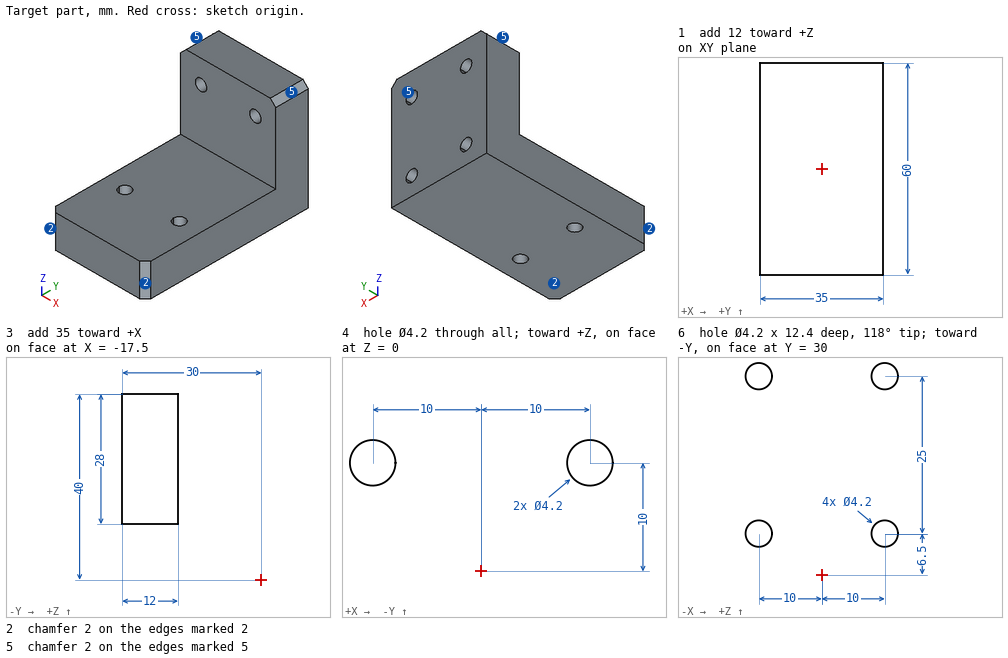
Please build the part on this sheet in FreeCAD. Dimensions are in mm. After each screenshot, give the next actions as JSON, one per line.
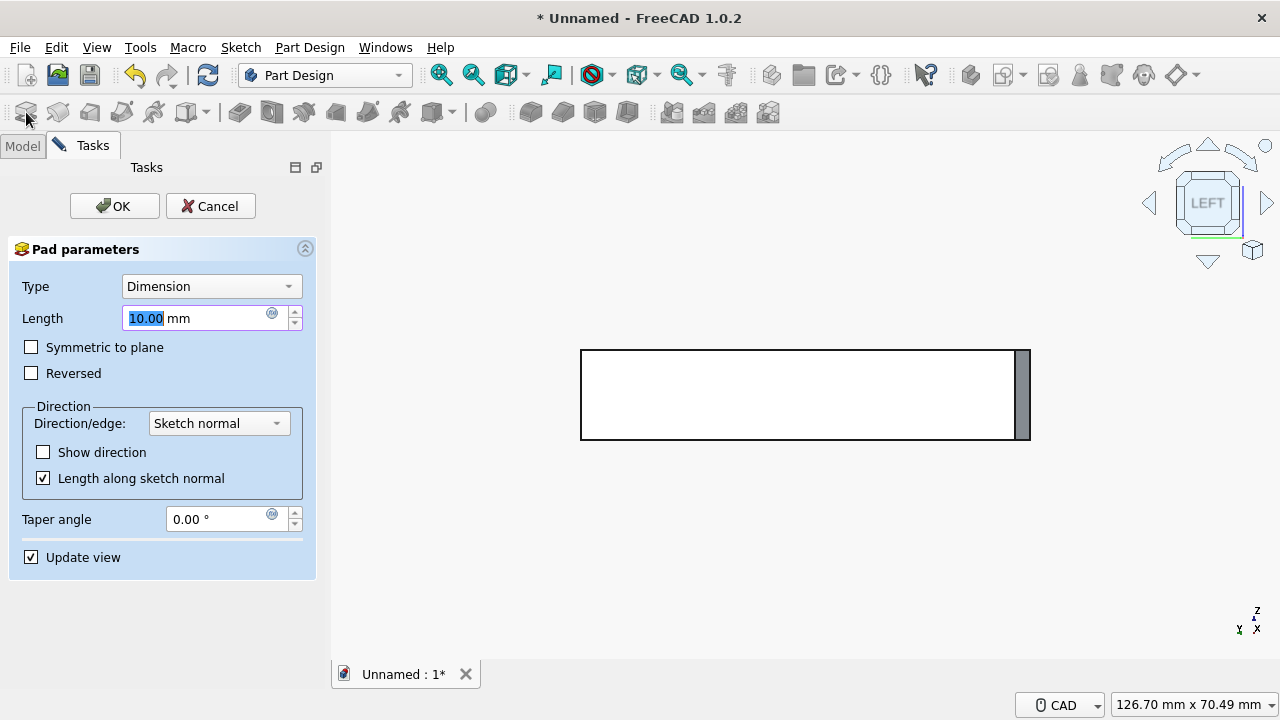
{"action": "type", "text": "35"}
{"action": "key", "text": "Tab"}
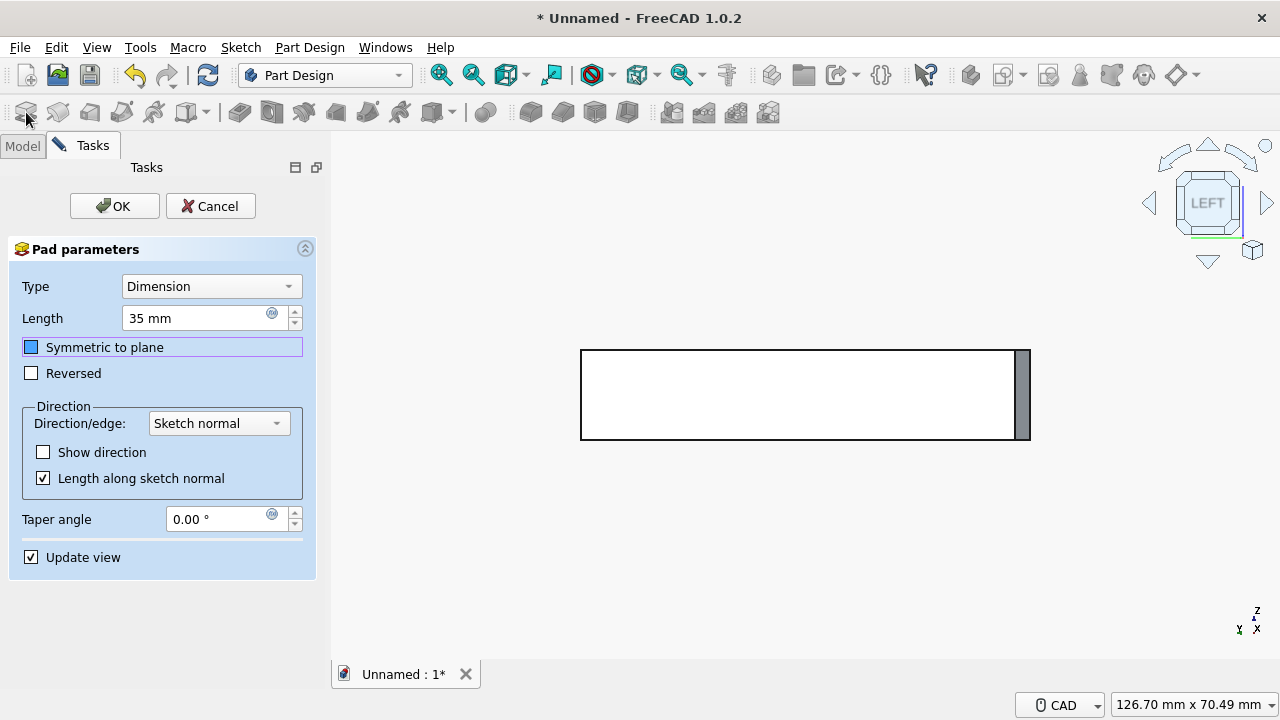
{"action": "left_click", "coordinate": [30, 373]}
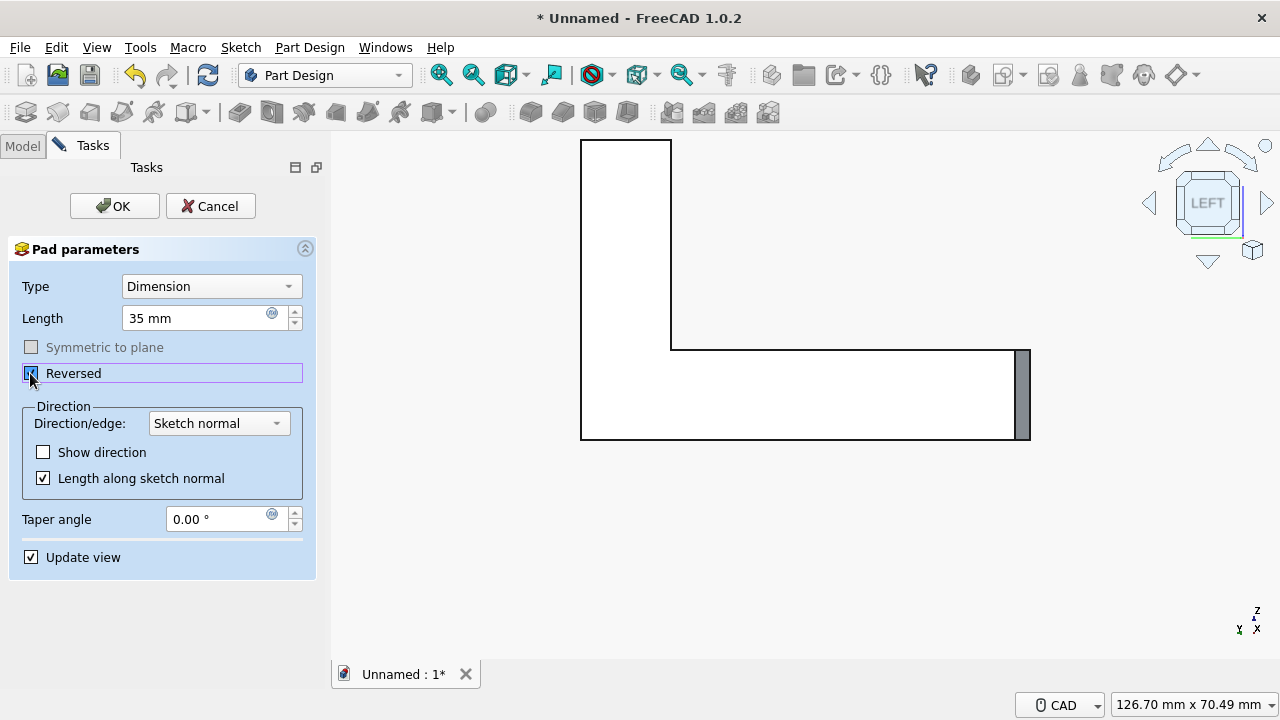
{"action": "left_click", "coordinate": [115, 206]}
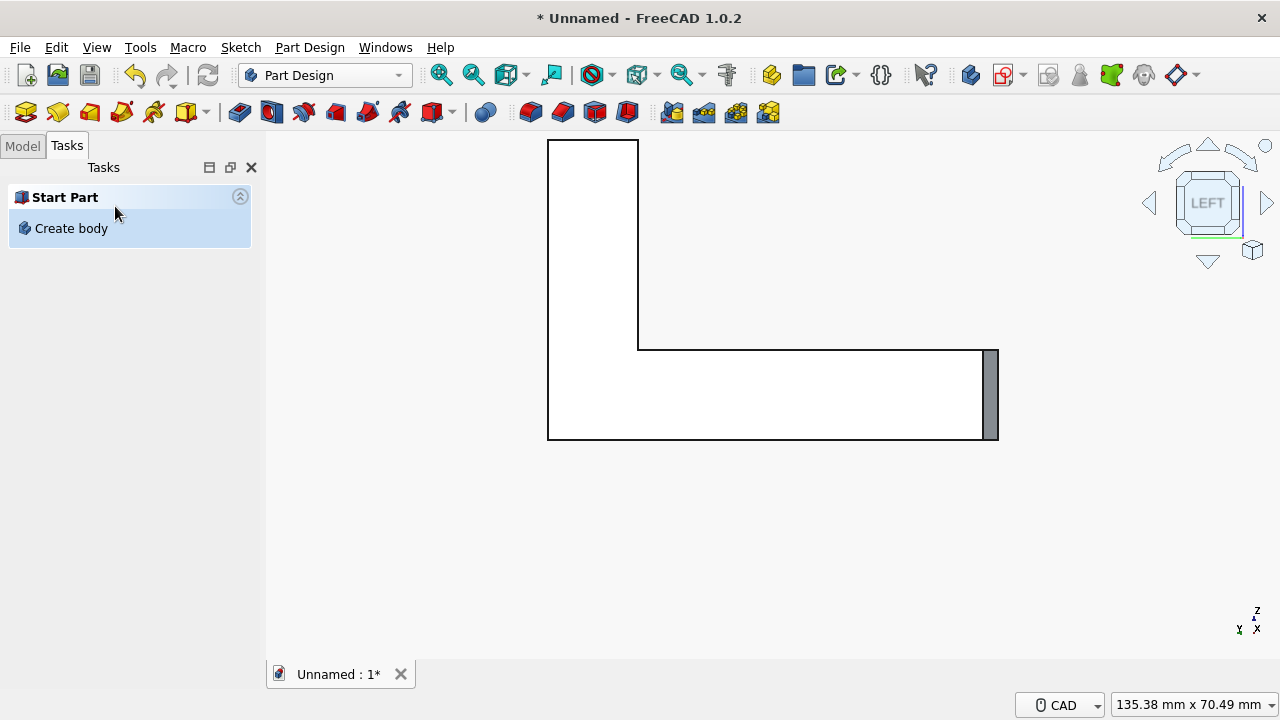
{"action": "key", "text": "5"}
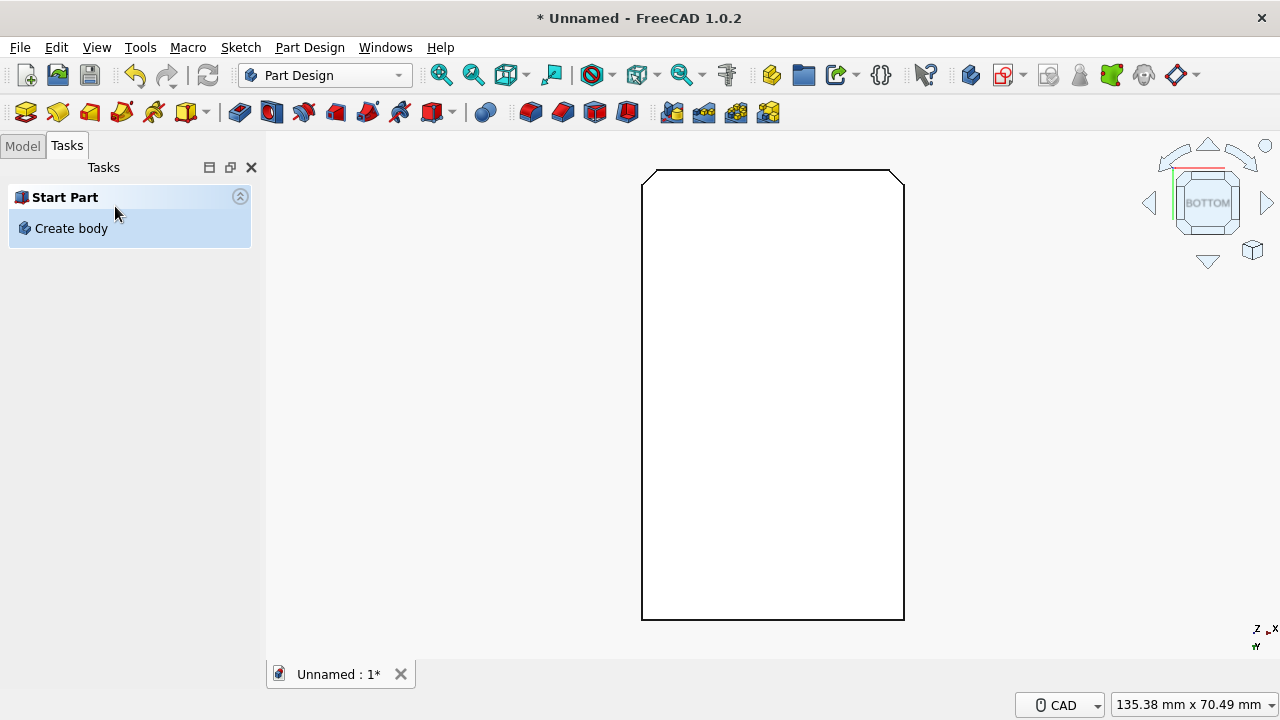
{"action": "left_click", "coordinate": [773, 458]}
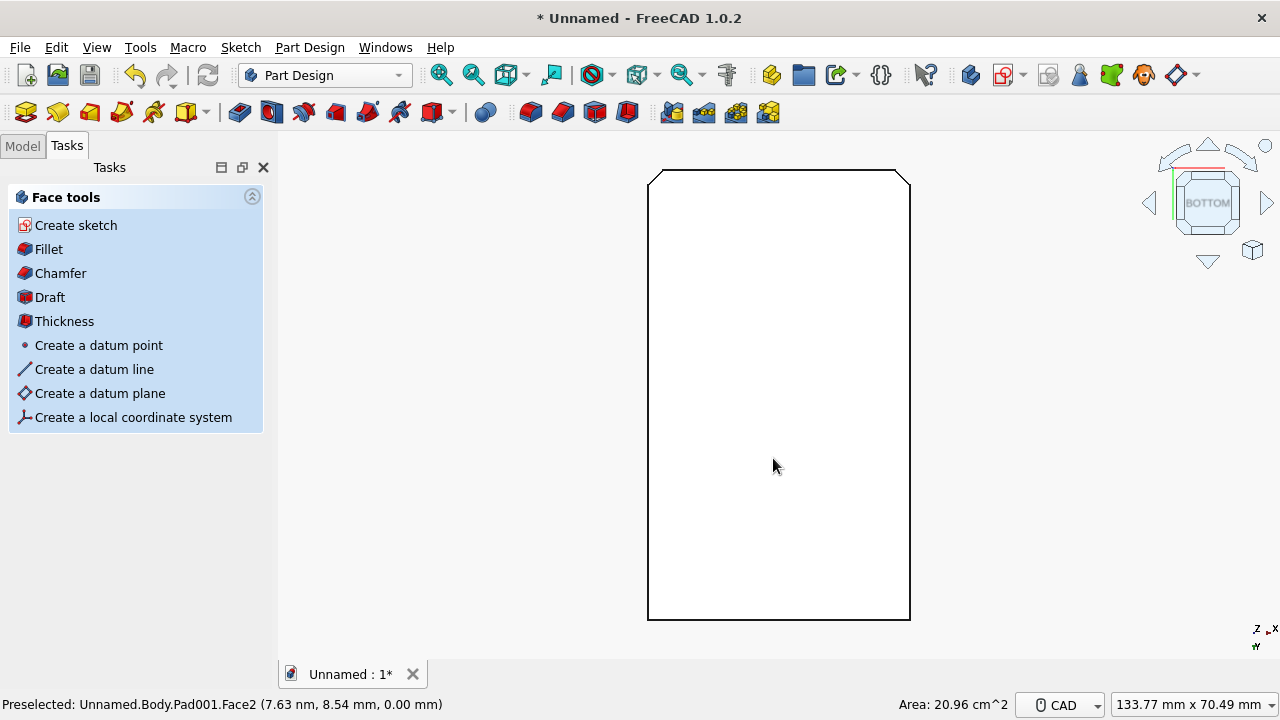
{"action": "left_click", "coordinate": [1004, 76]}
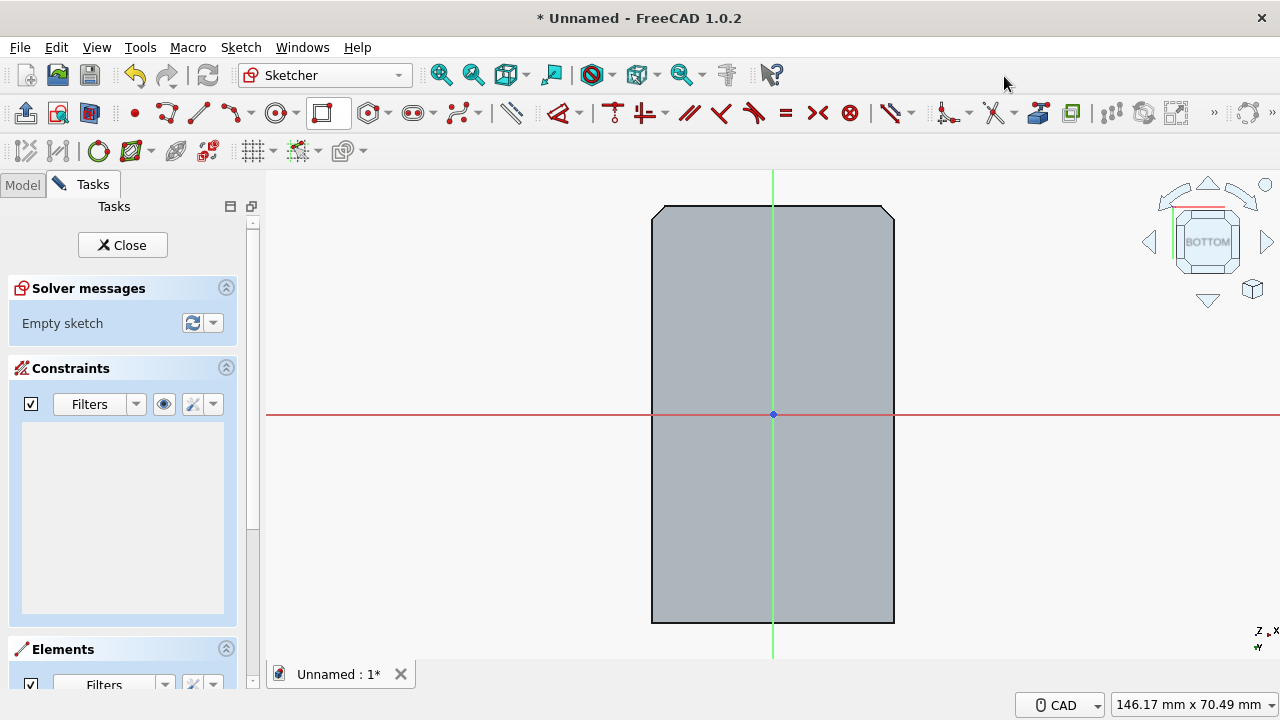
{"action": "scroll", "coordinate": [803, 354], "scroll_direction": "up", "scroll_amount": 6}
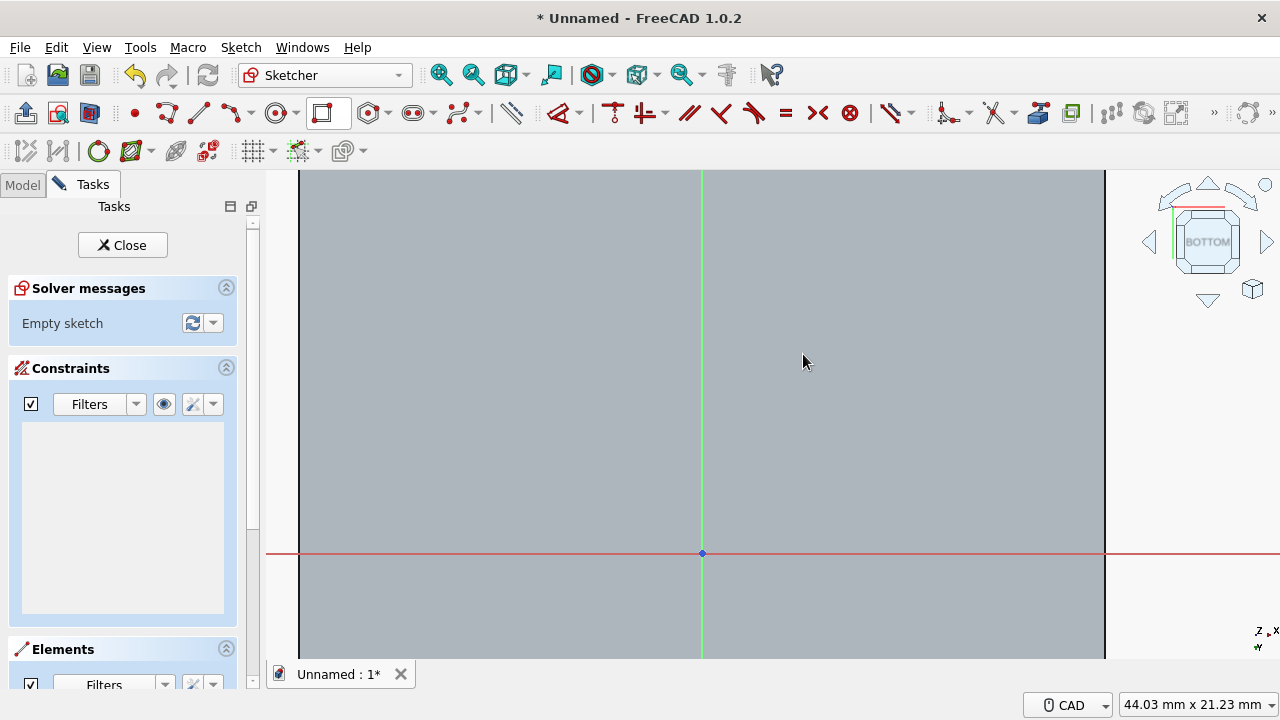
{"action": "left_click", "coordinate": [276, 114]}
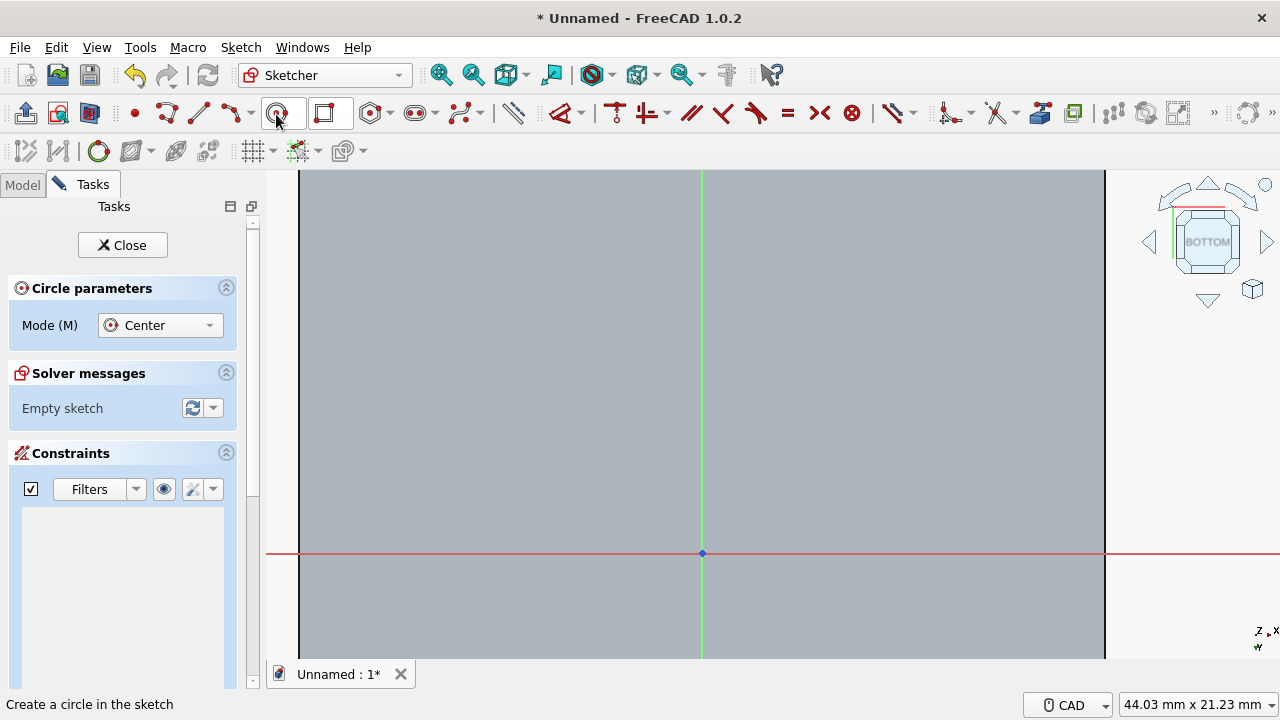
{"action": "left_click", "coordinate": [932, 324]}
{"action": "left_click", "coordinate": [967, 289]}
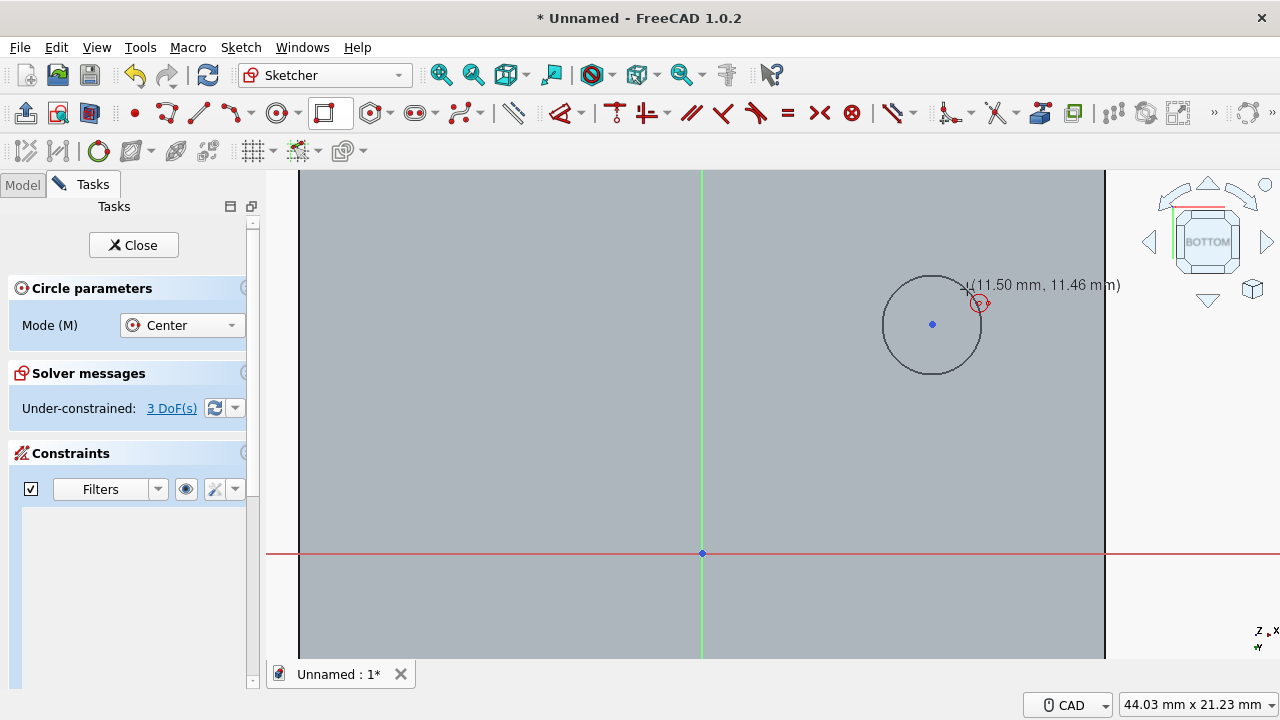
{"action": "left_click", "coordinate": [472, 324]}
{"action": "left_click", "coordinate": [506, 289]}
{"action": "key", "text": "Escape"}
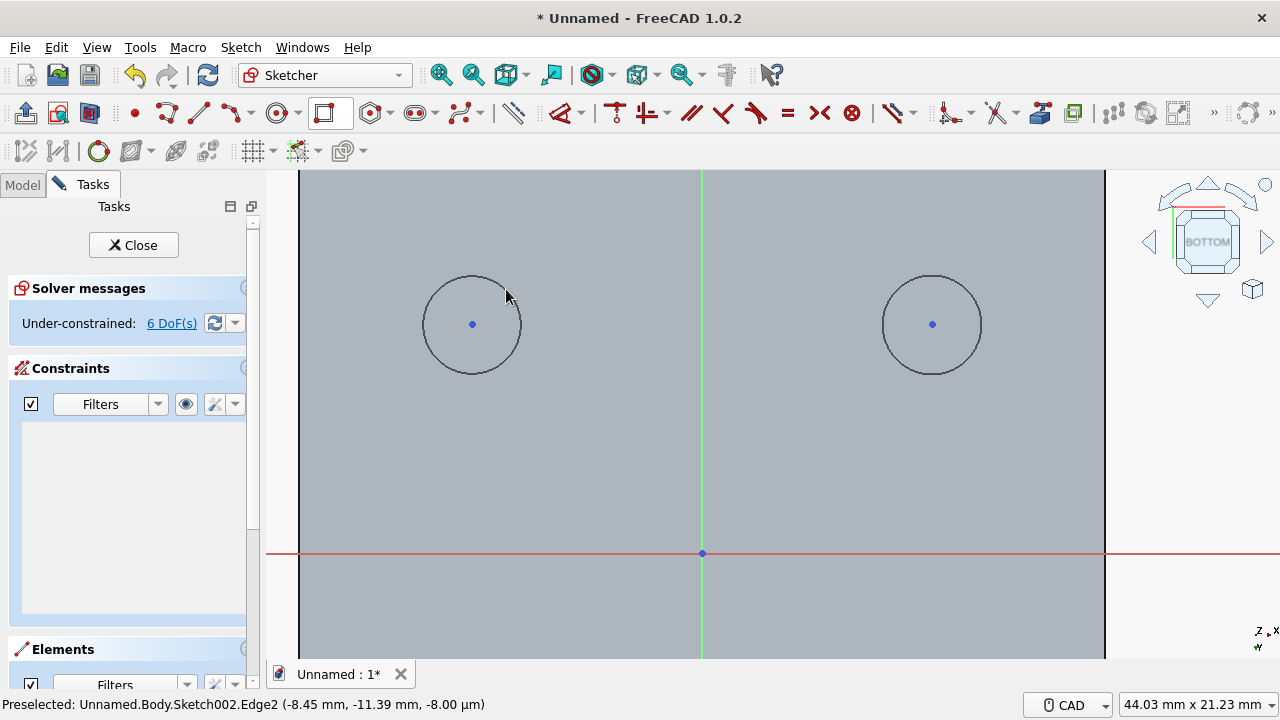
{"action": "left_click", "coordinate": [967, 290]}